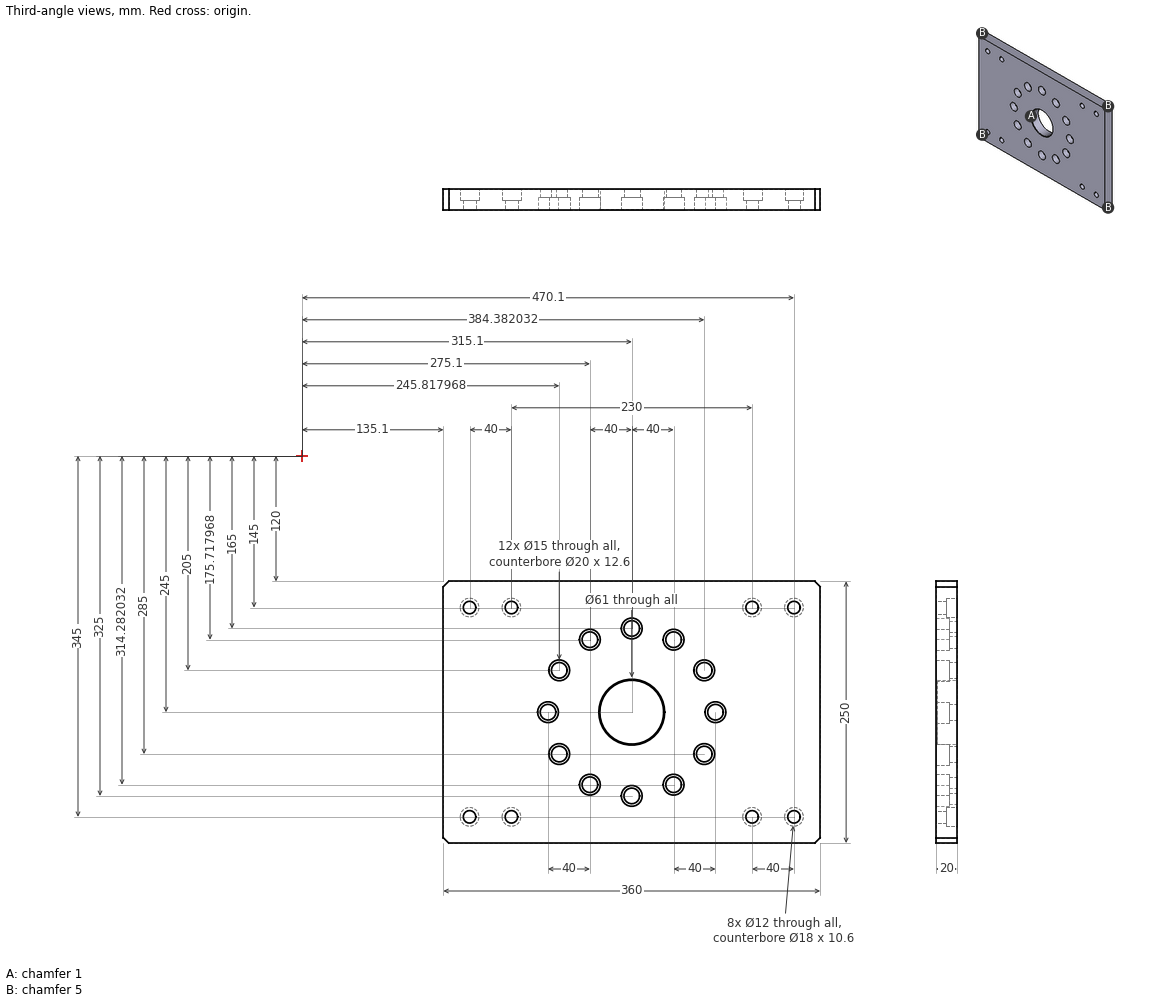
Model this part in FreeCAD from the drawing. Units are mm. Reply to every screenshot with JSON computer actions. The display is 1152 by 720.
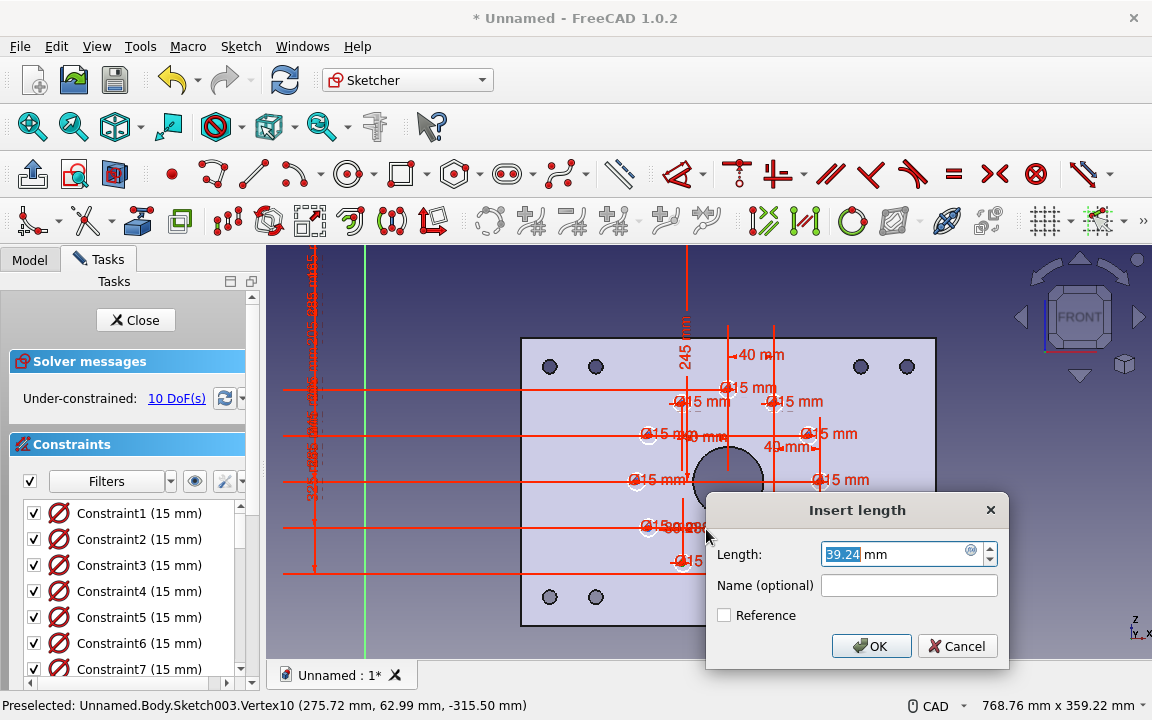
{"action": "type", "text": "40"}
{"action": "key", "text": "Return"}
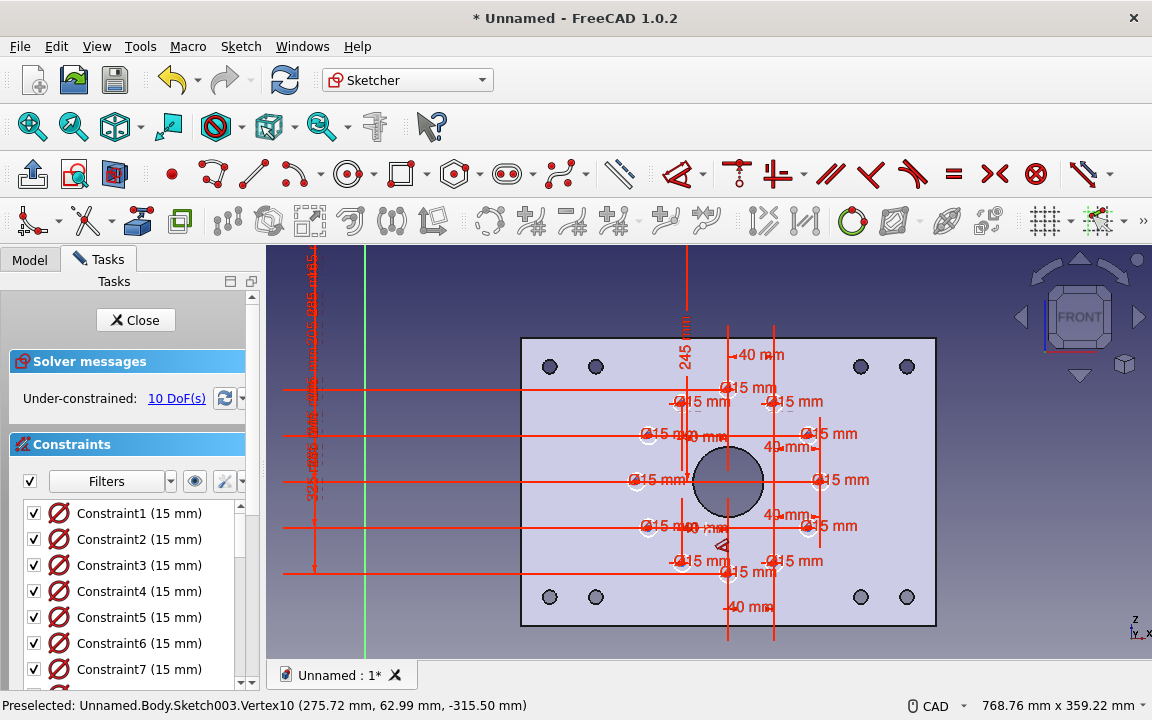
{"action": "left_click", "coordinate": [682, 404]}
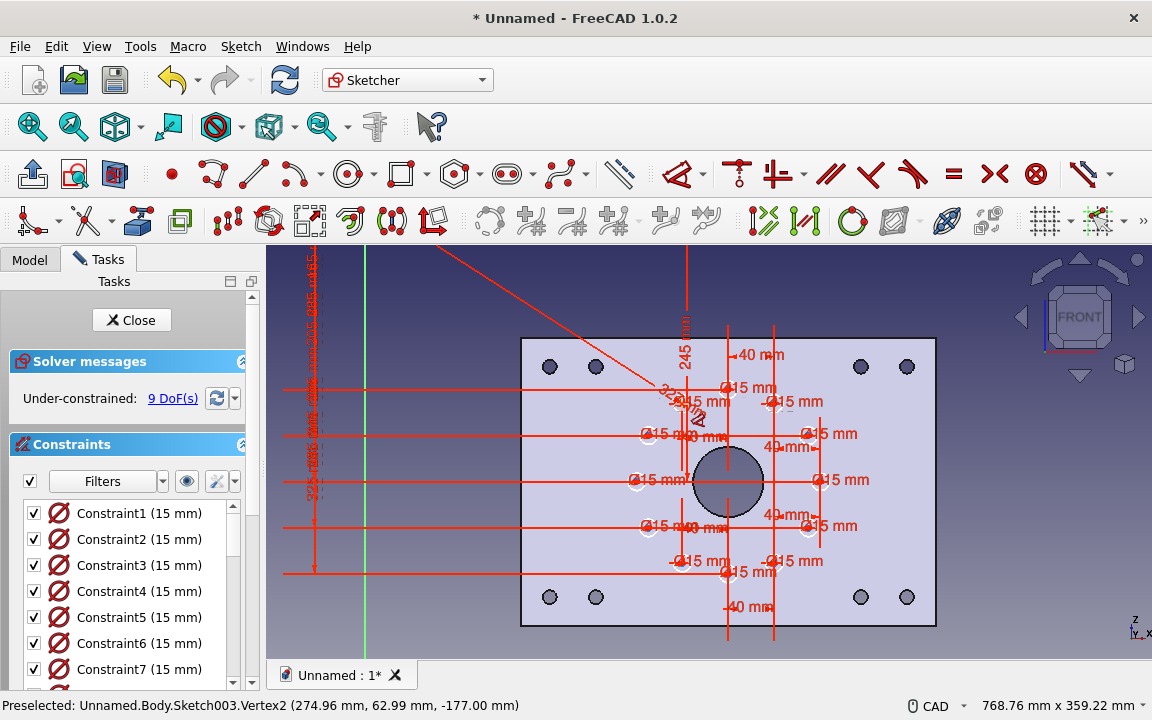
{"action": "left_click", "coordinate": [637, 482]}
{"action": "left_click", "coordinate": [659, 370]}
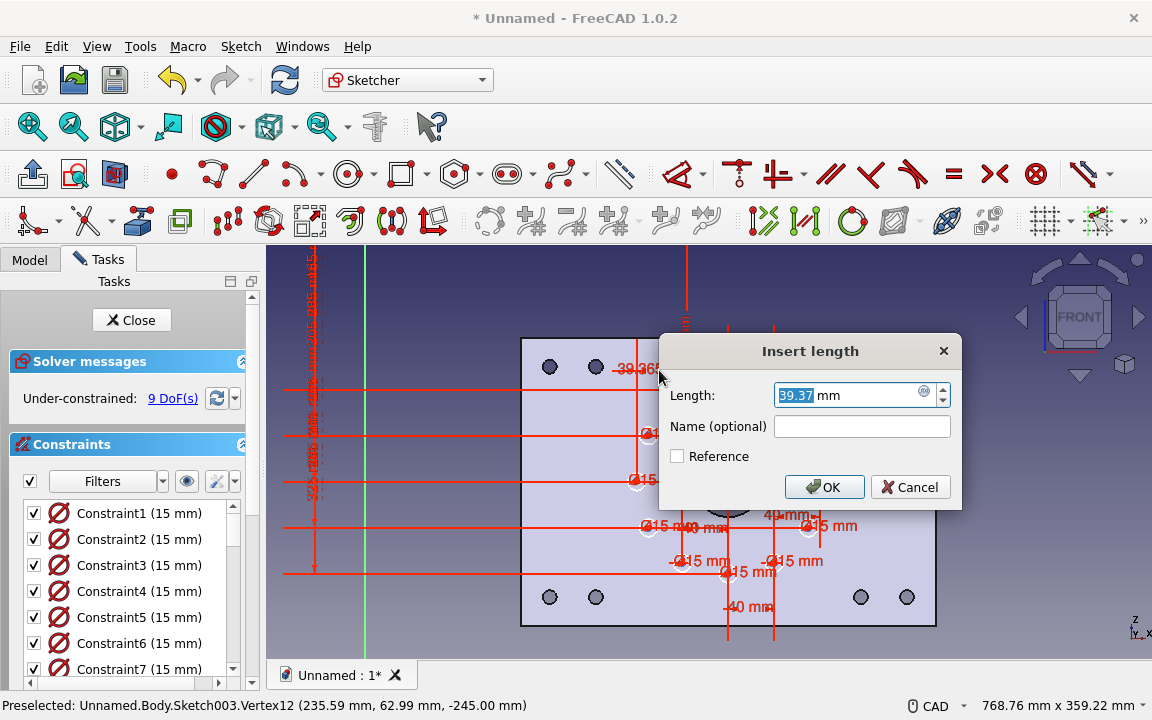
{"action": "type", "text": "40"}
{"action": "key", "text": "Return"}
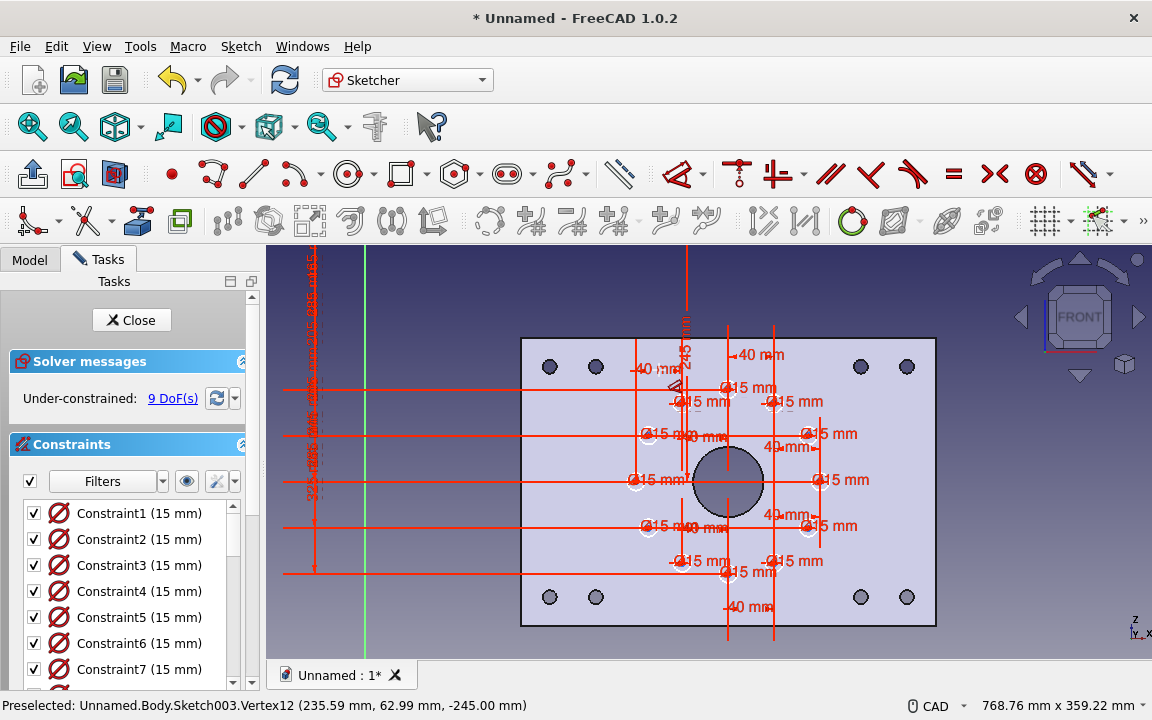
{"action": "left_click", "coordinate": [682, 404]}
{"action": "left_click", "coordinate": [524, 438]}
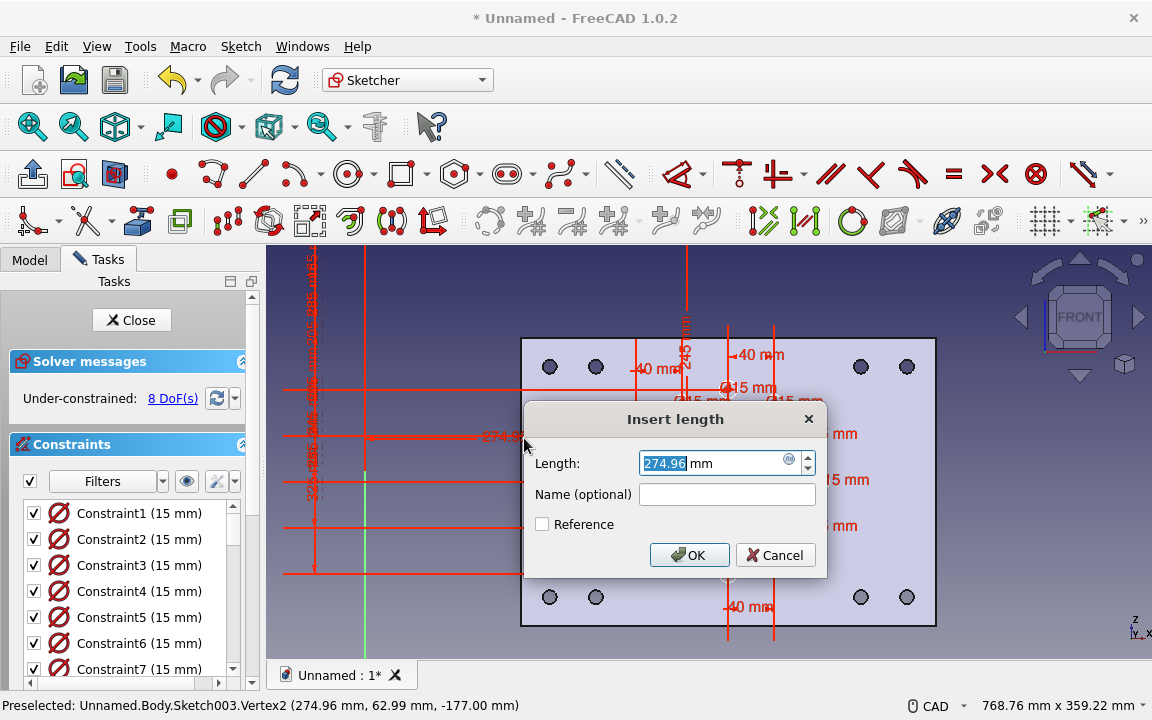
{"action": "type", "text": "275.1"}
{"action": "key", "text": "Return"}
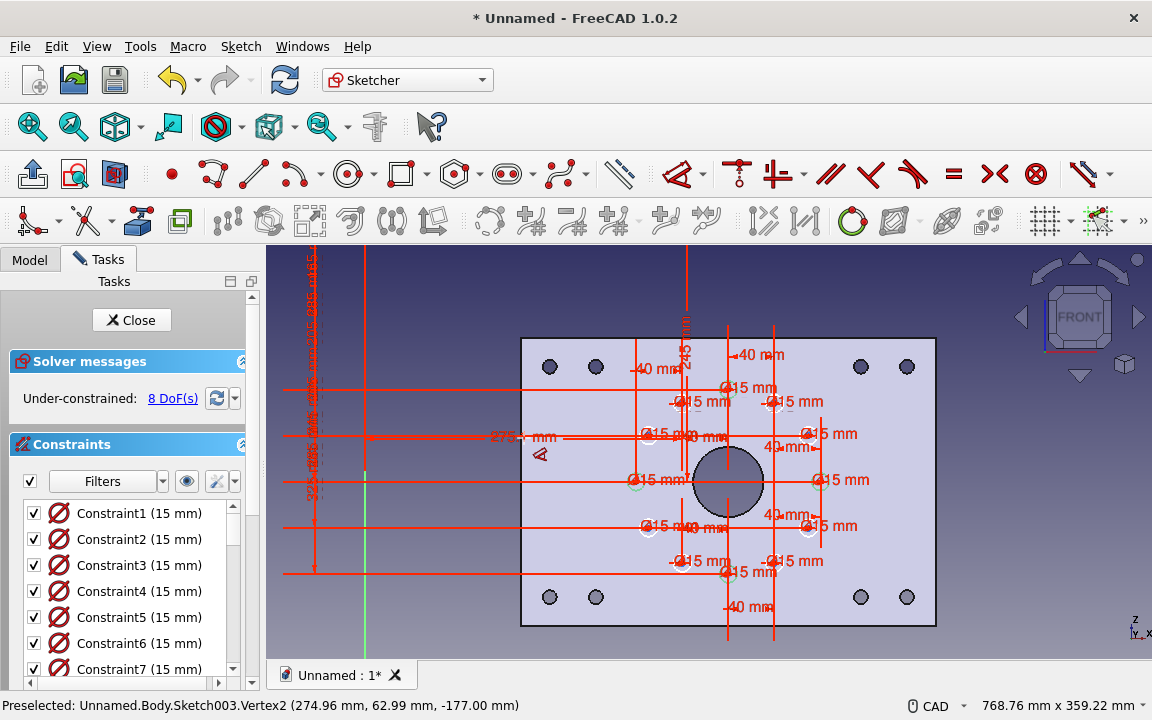
{"action": "left_click", "coordinate": [649, 436]}
{"action": "left_click", "coordinate": [507, 470]}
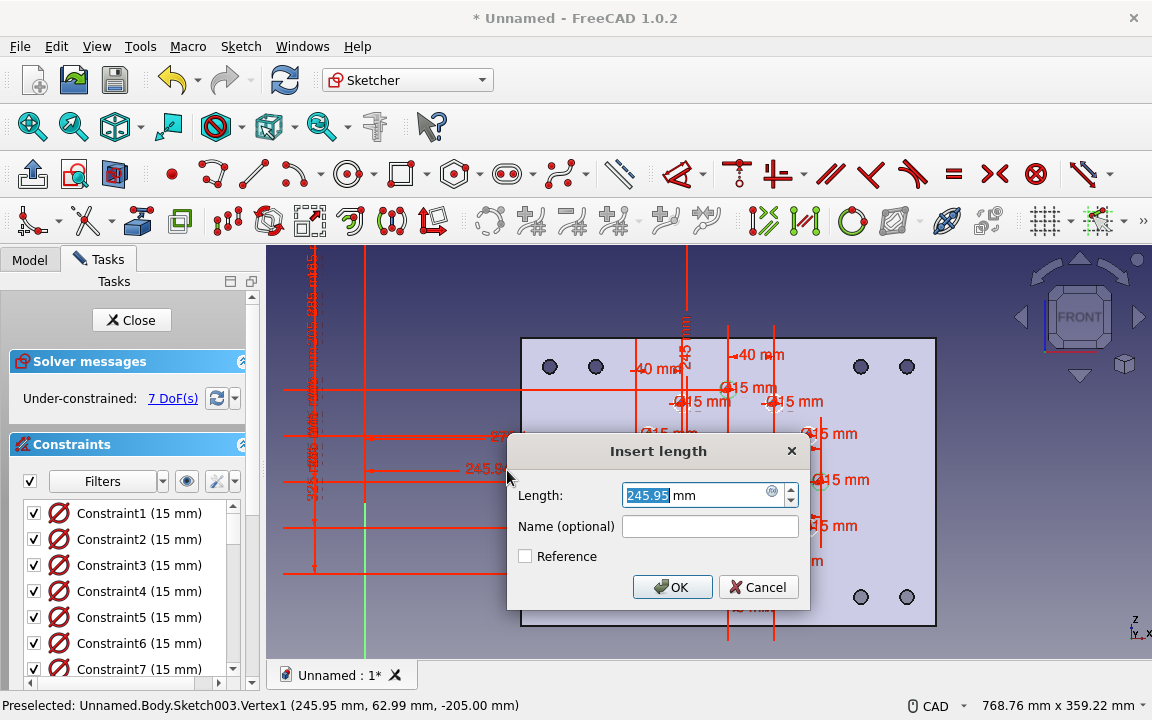
{"action": "type", "text": "245.817968"}
{"action": "key", "text": "Return"}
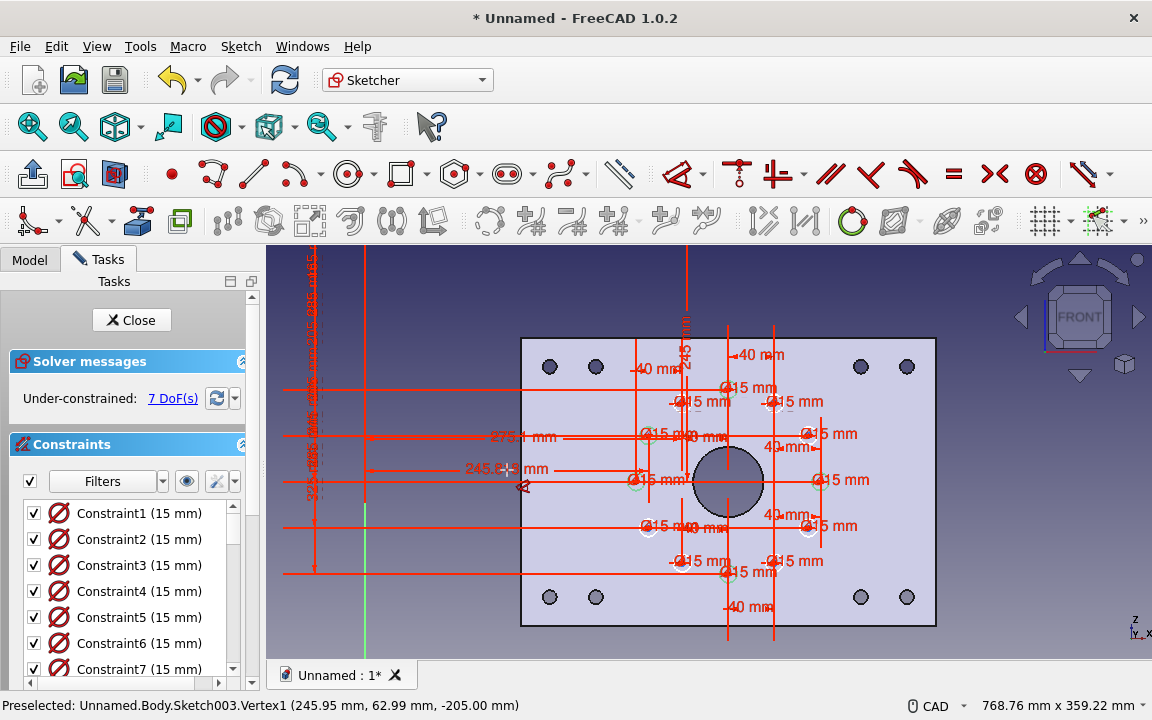
{"action": "left_click", "coordinate": [682, 404]}
{"action": "left_click", "coordinate": [716, 308]}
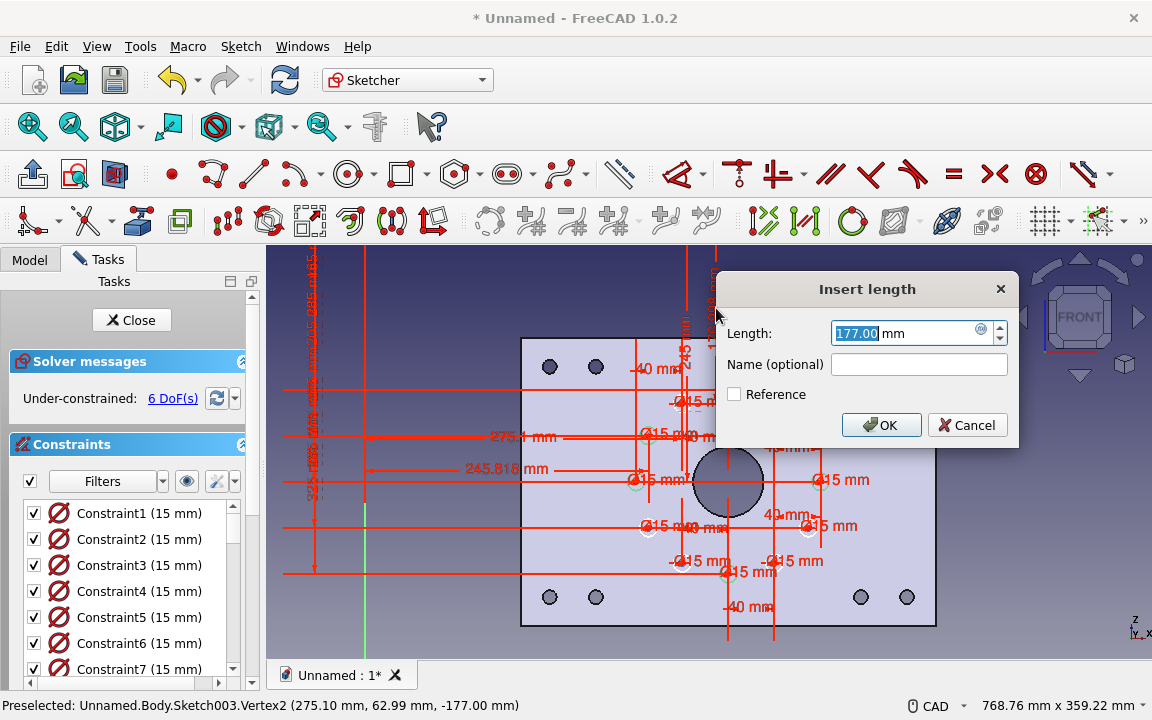
{"action": "type", "text": "175.717968"}
{"action": "key", "text": "Return"}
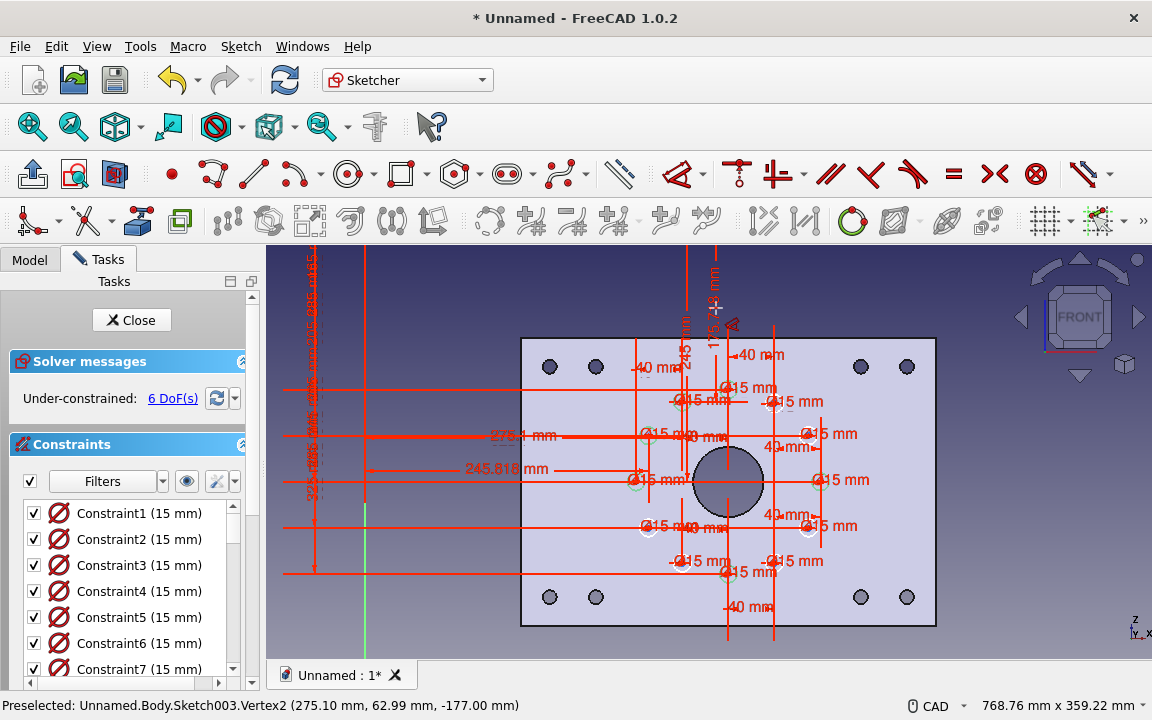
{"action": "left_click", "coordinate": [774, 404]}
{"action": "left_click", "coordinate": [808, 308]}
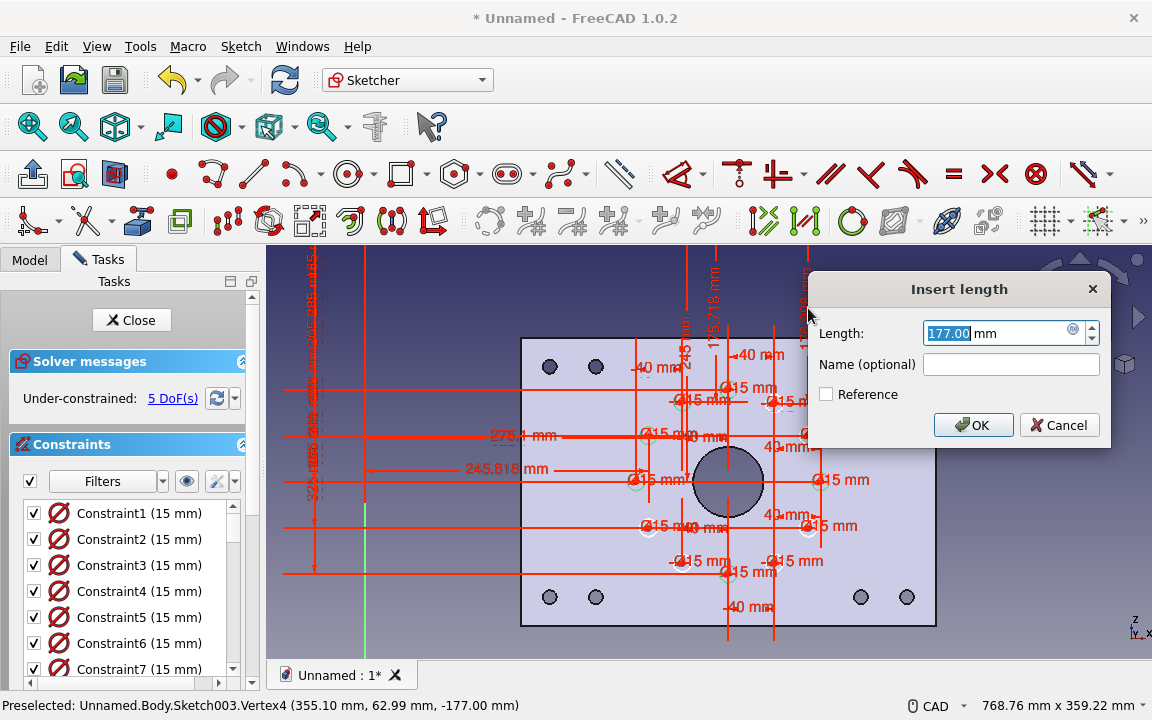
{"action": "type", "text": "175.717968"}
{"action": "key", "text": "Return"}